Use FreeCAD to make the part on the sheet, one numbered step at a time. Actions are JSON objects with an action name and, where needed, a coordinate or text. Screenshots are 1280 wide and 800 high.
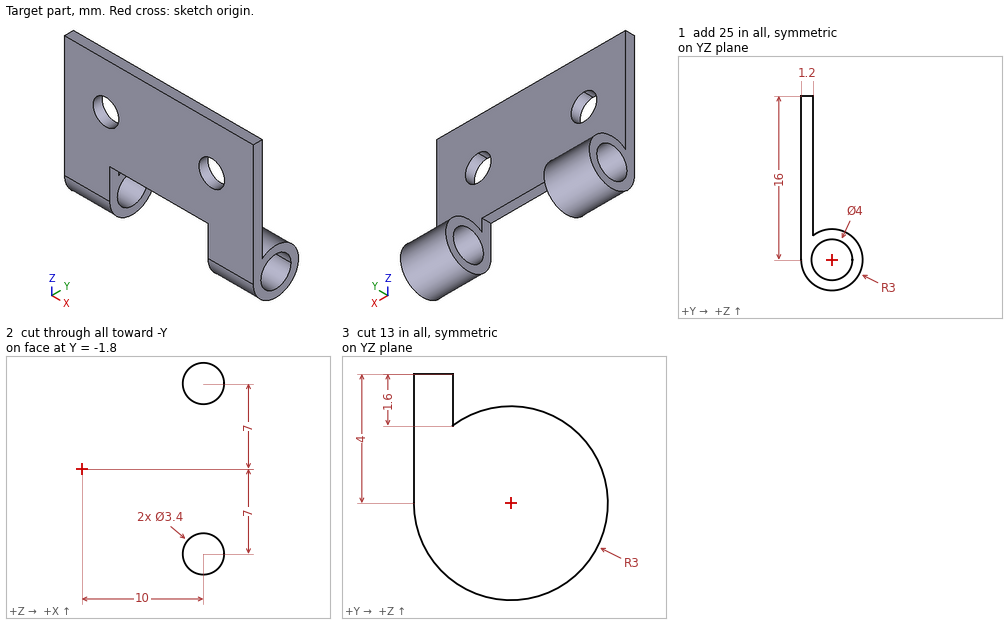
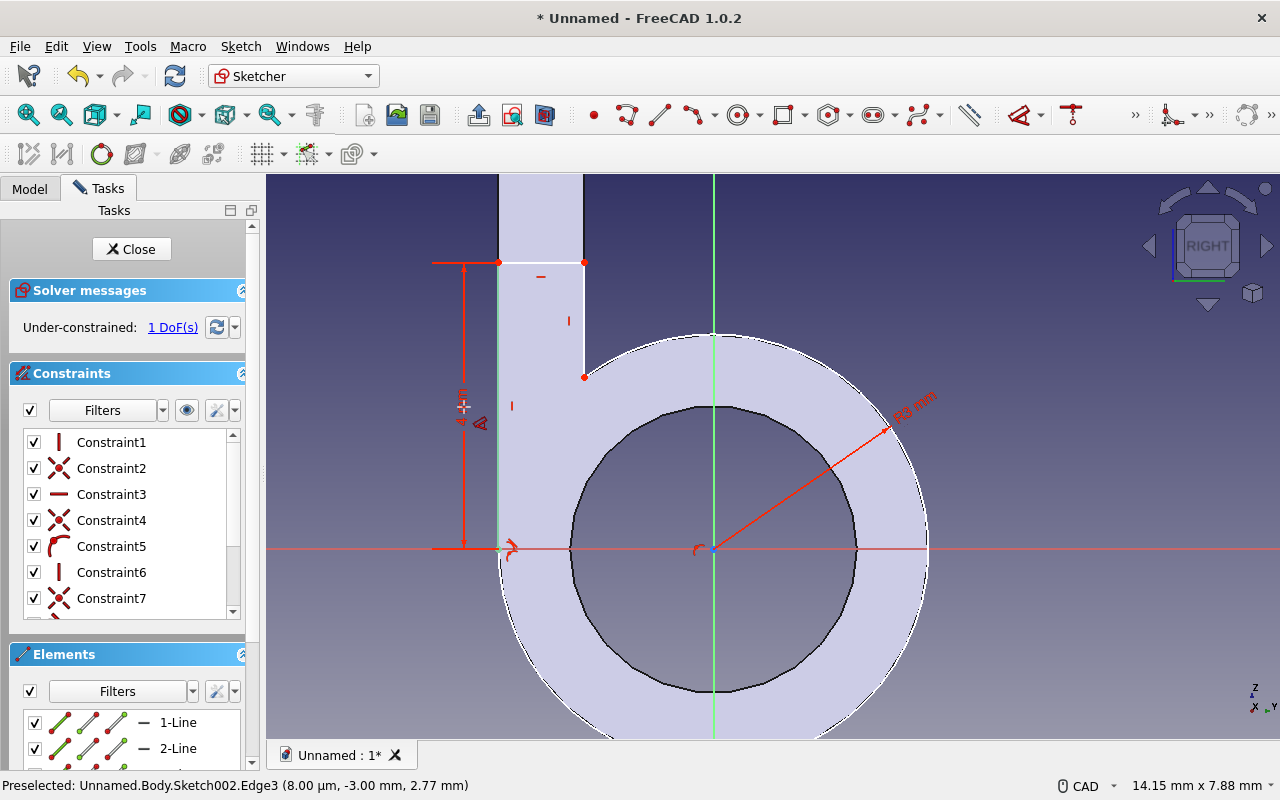
{"action": "left_click", "coordinate": [584, 343]}
{"action": "left_click", "coordinate": [550, 320]}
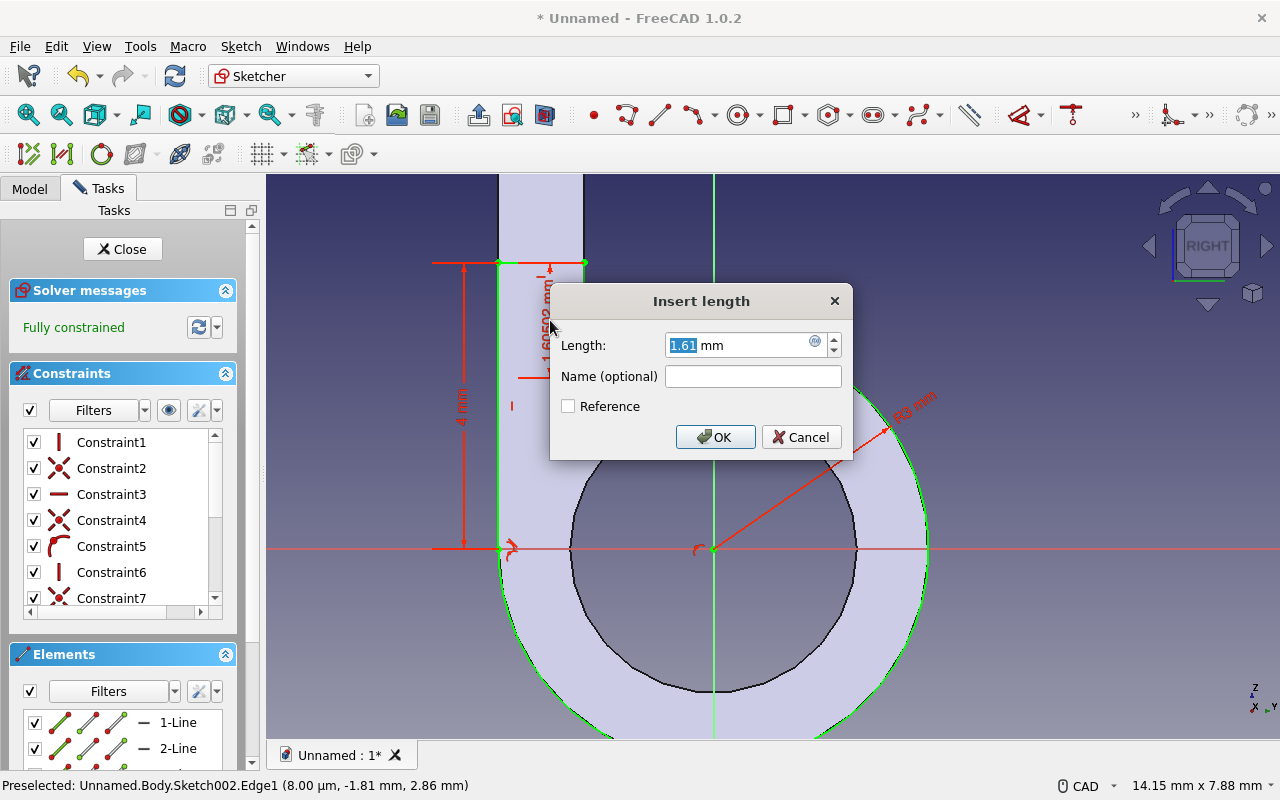
{"action": "type", "text": "1.6"}
{"action": "key", "text": "Return"}
{"action": "key", "text": "Escape"}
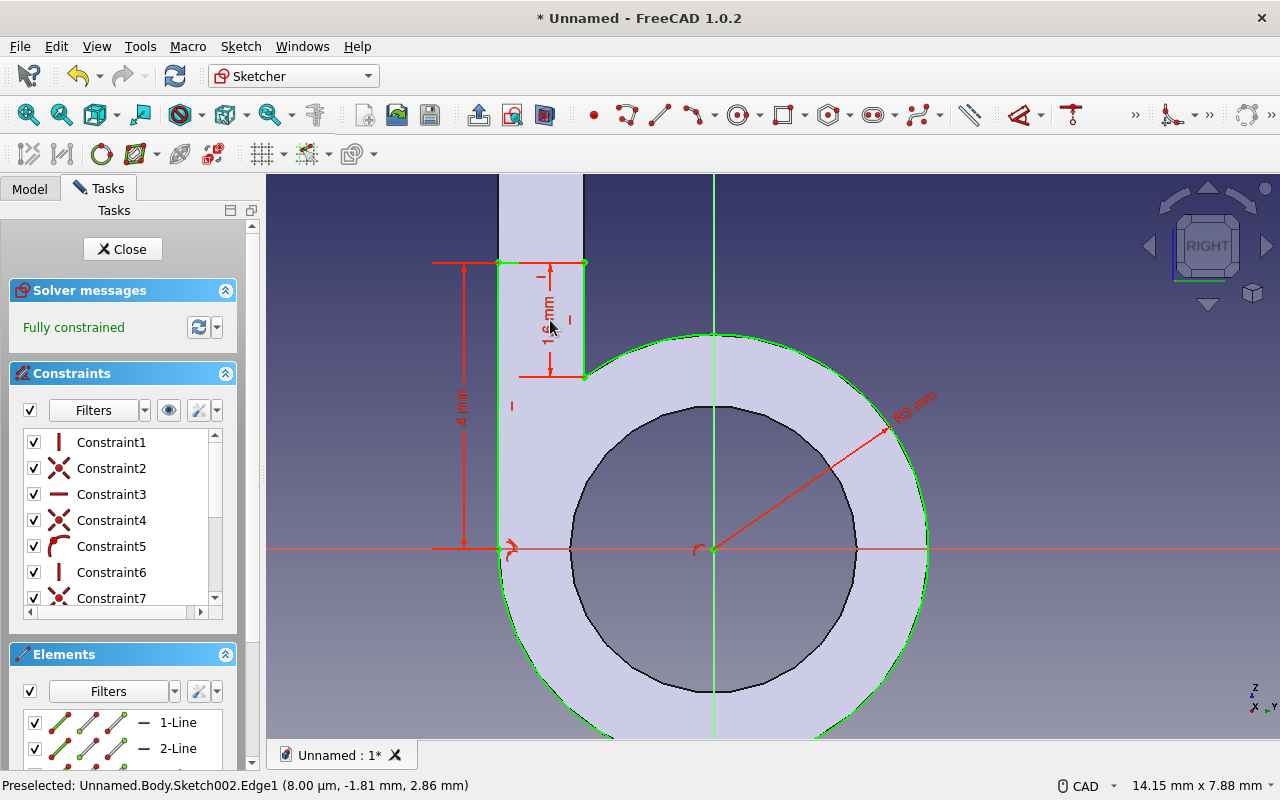
{"action": "left_click", "coordinate": [123, 249]}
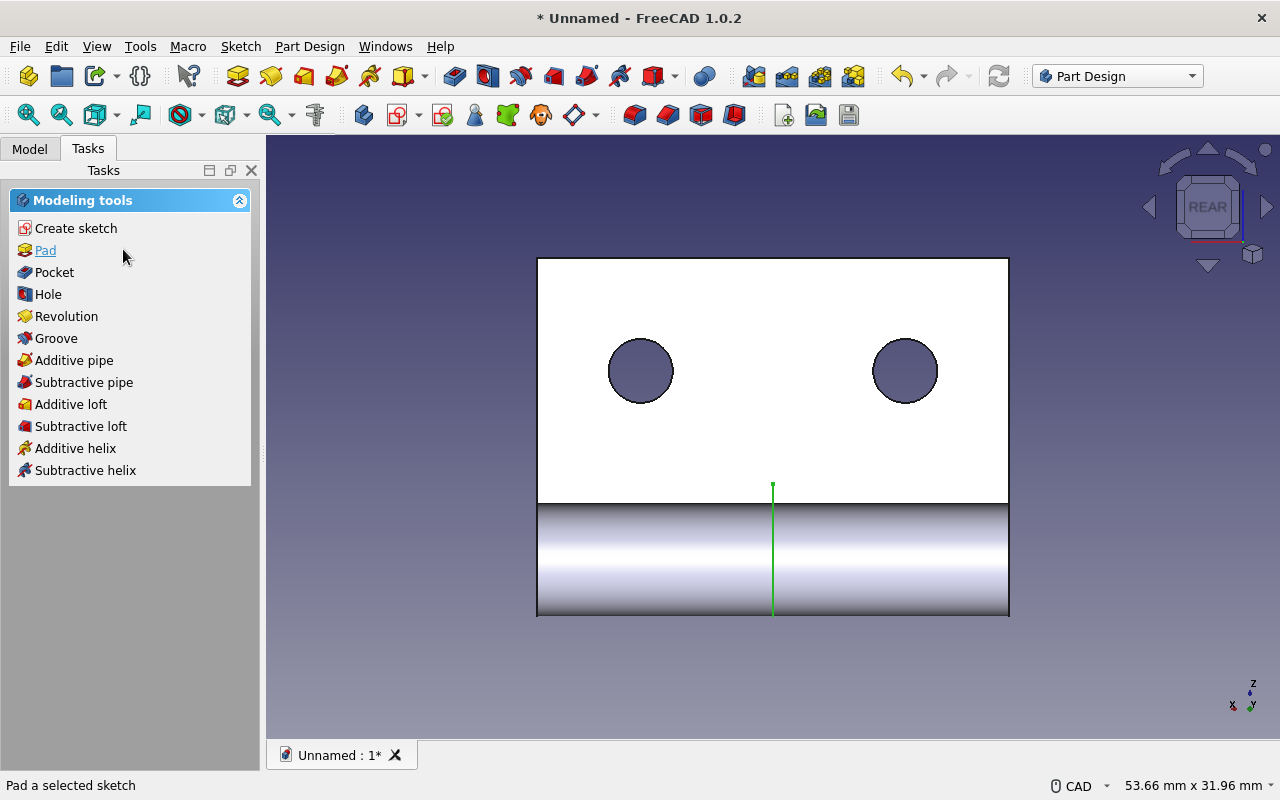
{"action": "left_click", "coordinate": [455, 76]}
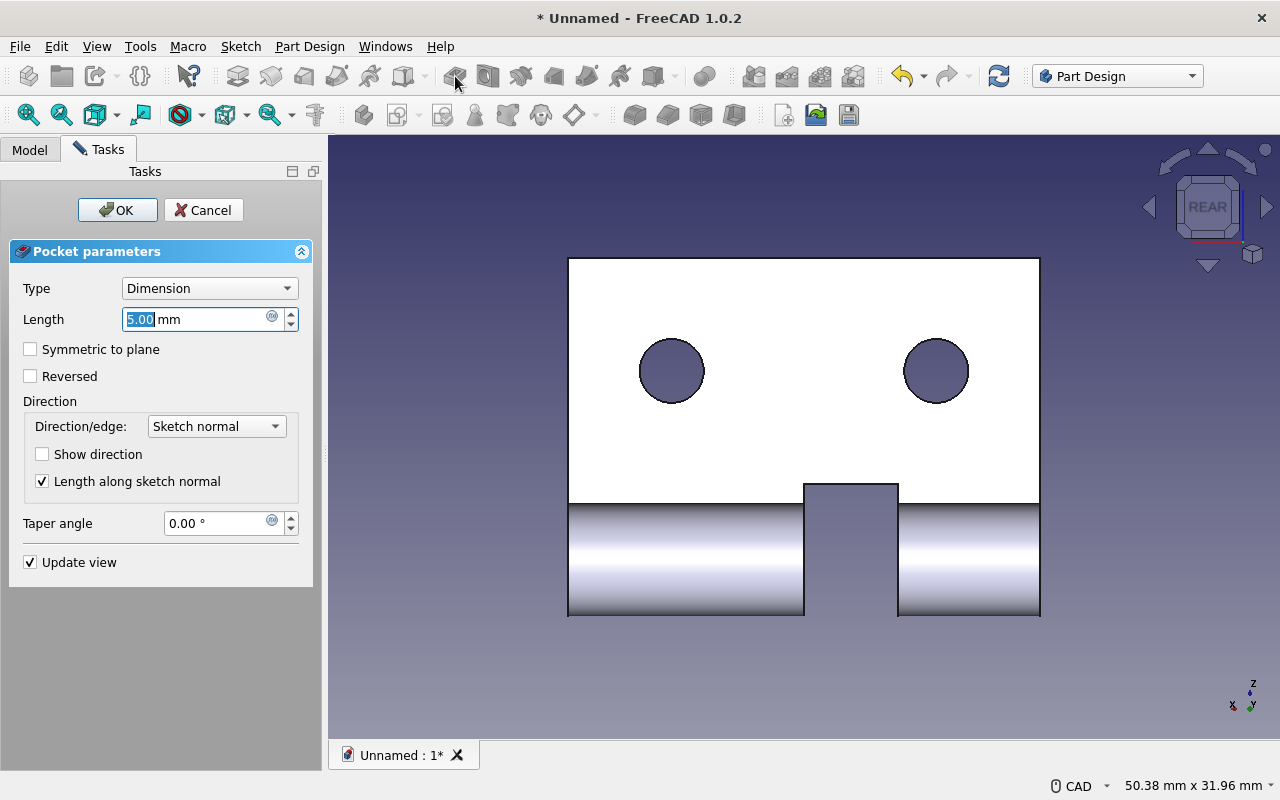
{"action": "type", "text": "13"}
{"action": "key", "text": "Tab"}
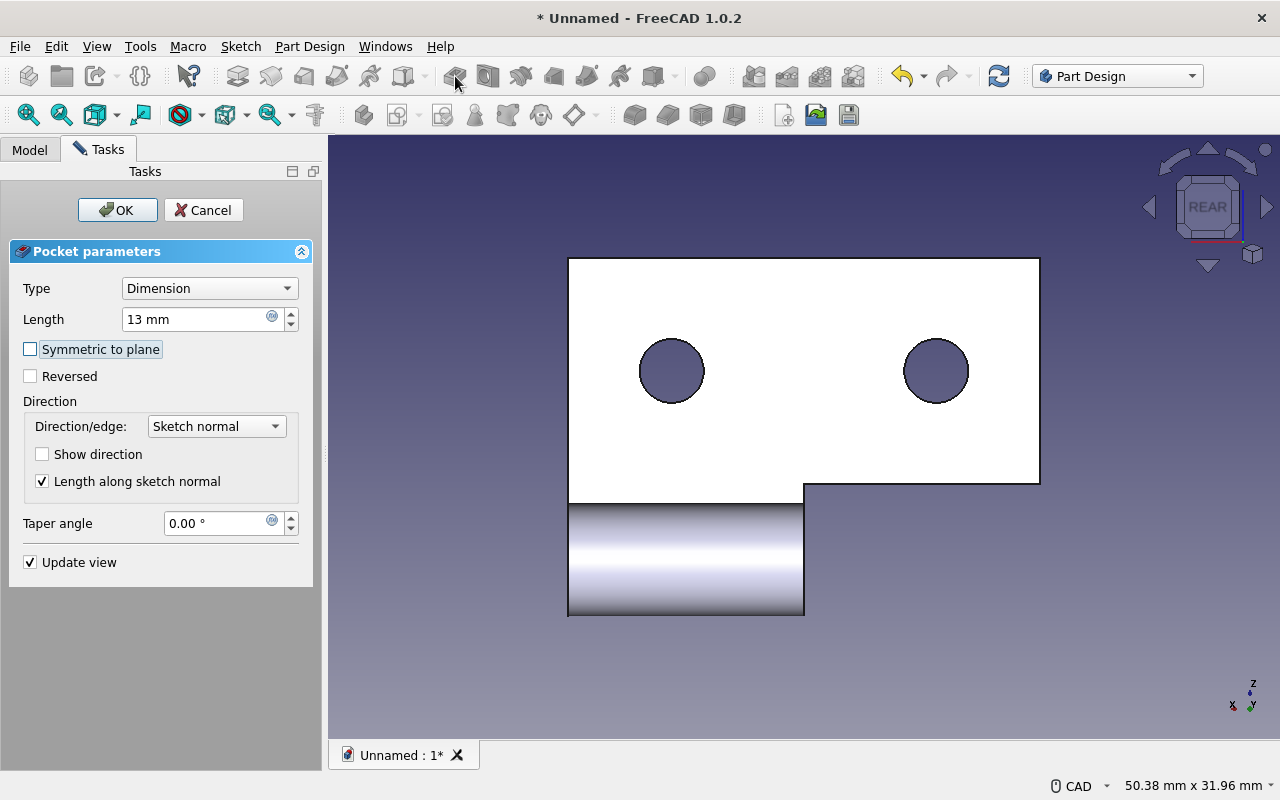
{"action": "left_click", "coordinate": [31, 349]}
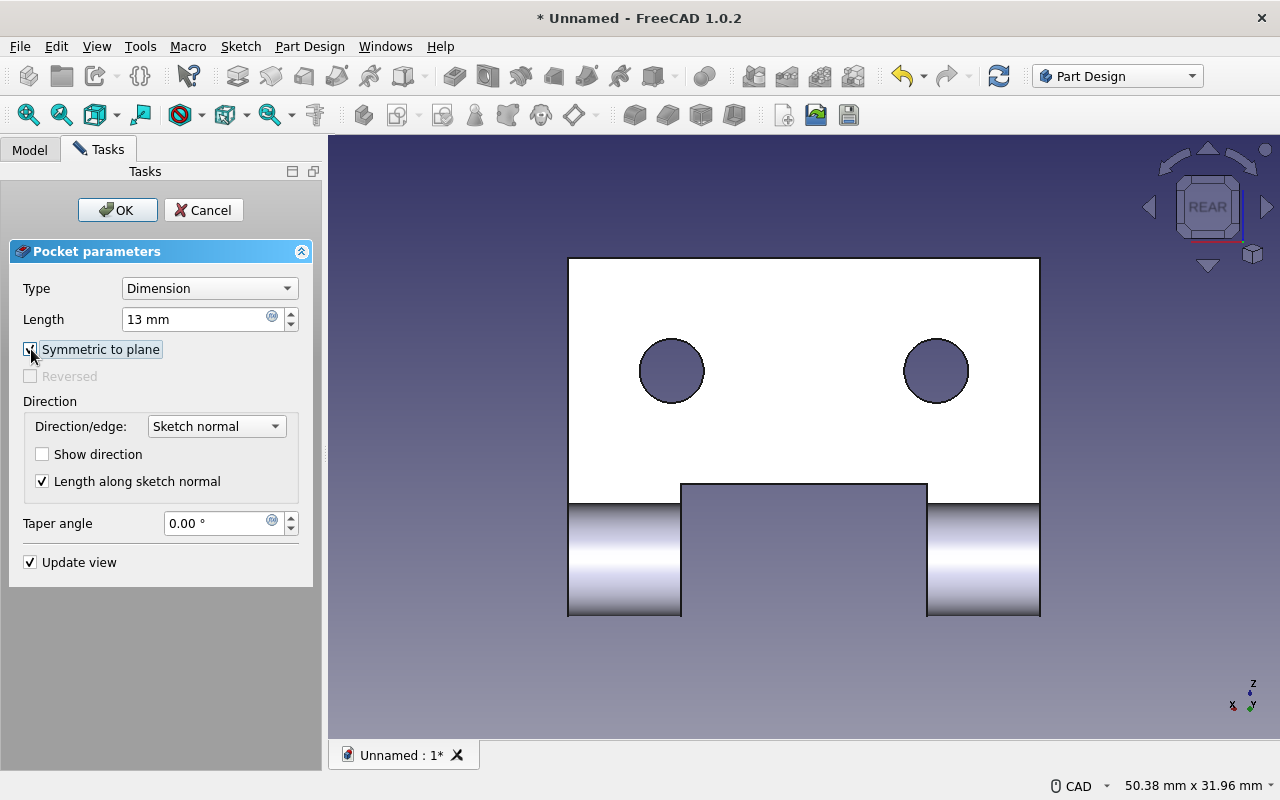
{"action": "left_click", "coordinate": [118, 210]}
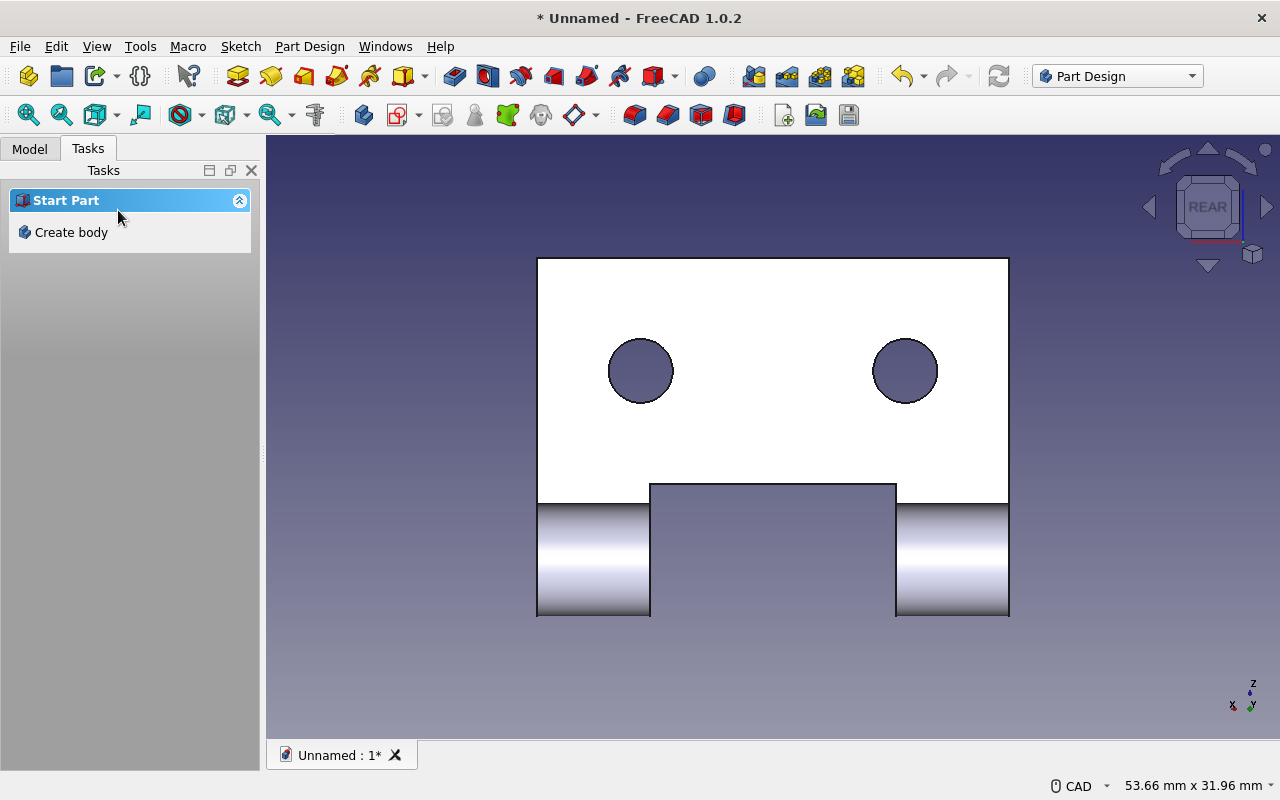
{"action": "key", "text": "0"}